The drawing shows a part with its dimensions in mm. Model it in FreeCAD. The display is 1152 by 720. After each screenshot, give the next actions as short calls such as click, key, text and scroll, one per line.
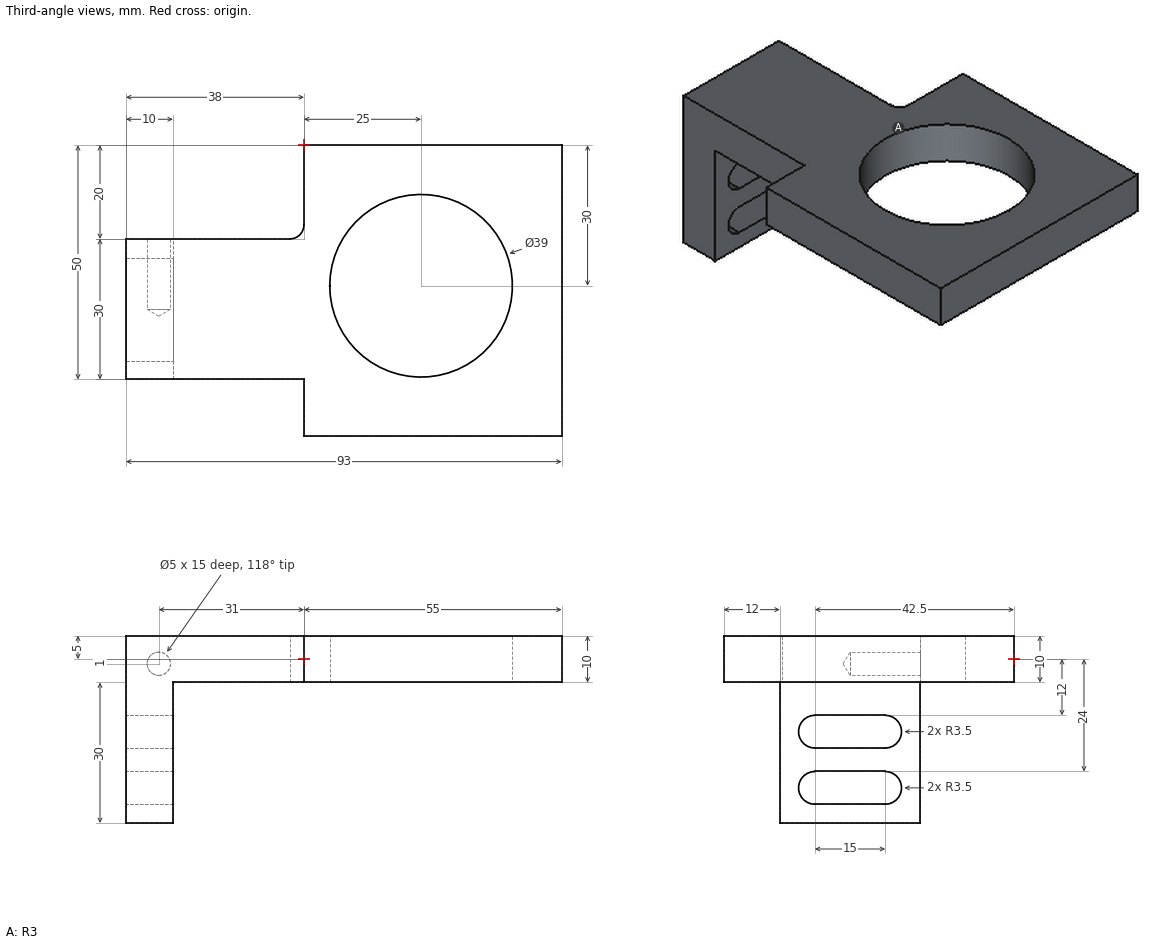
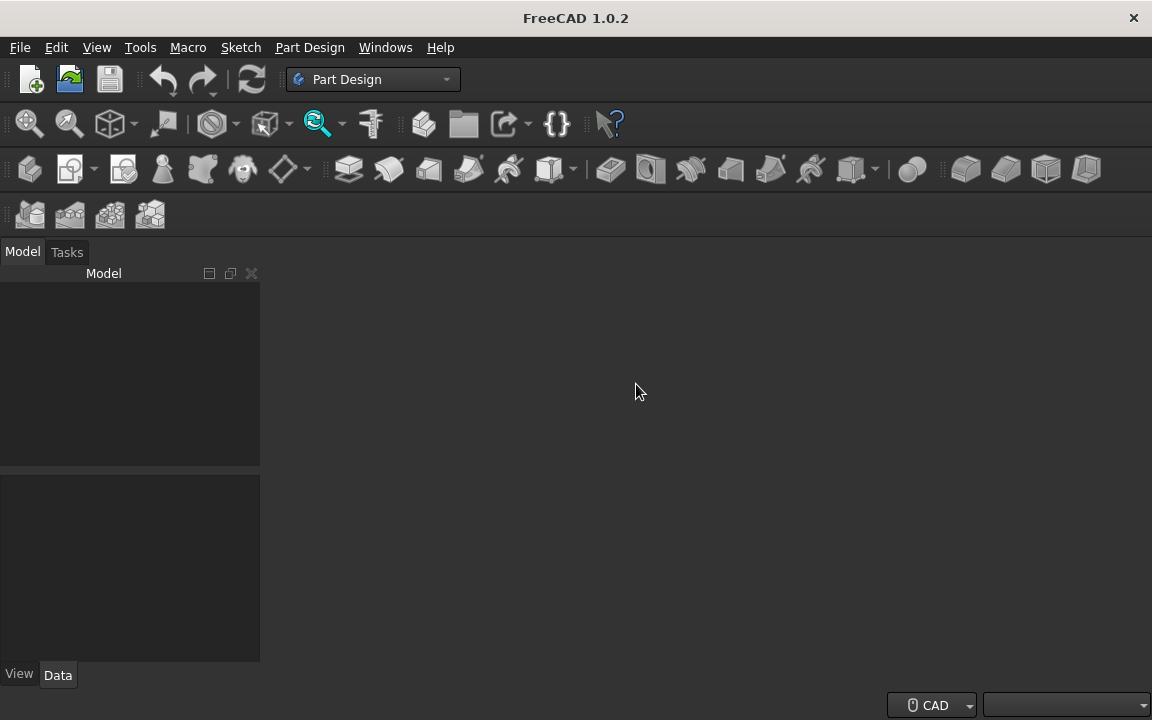
key(ctrl+n)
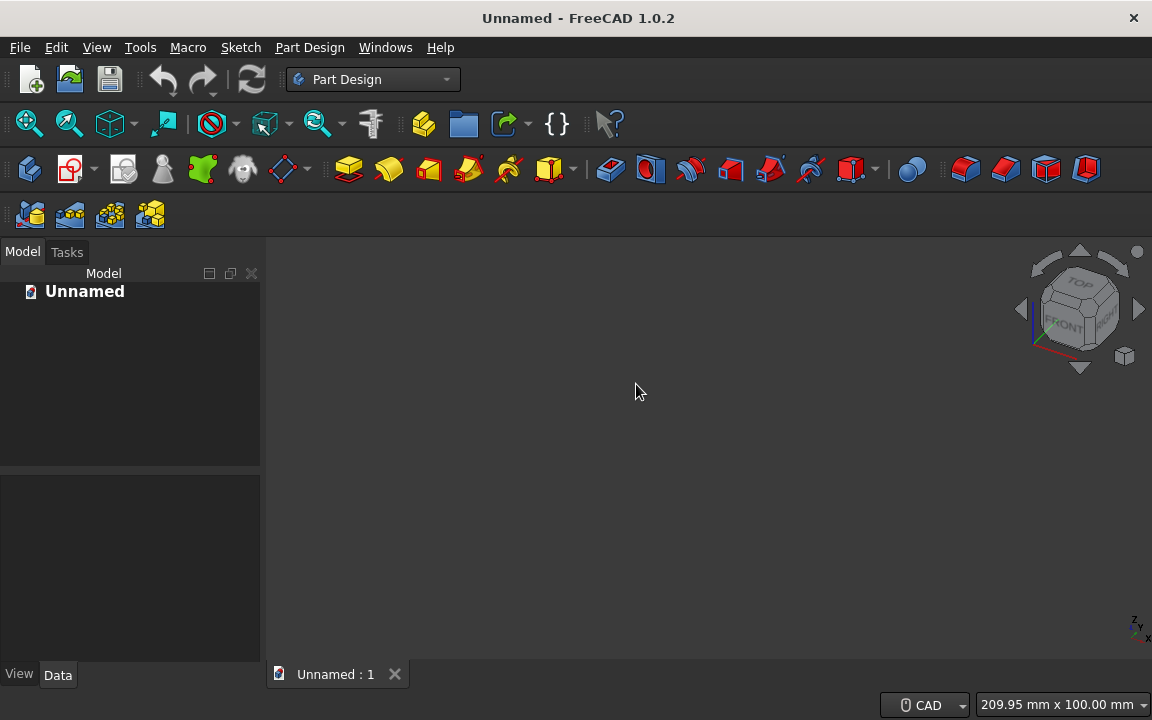
click(70, 170)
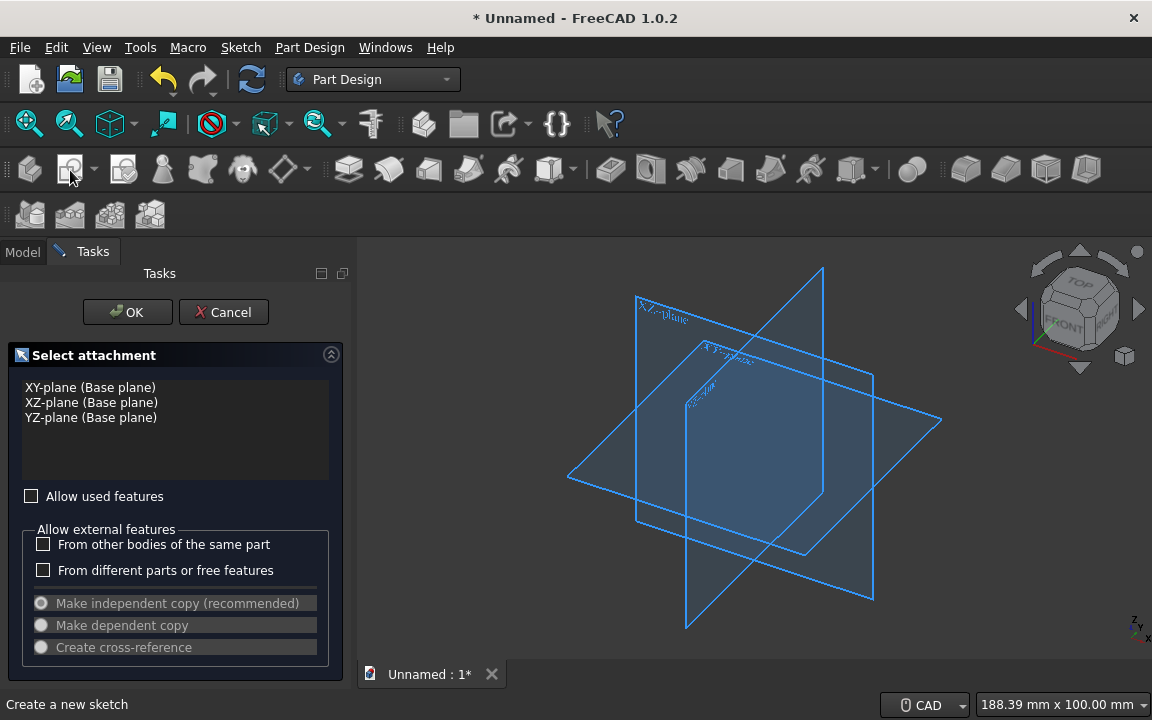
click(82, 388)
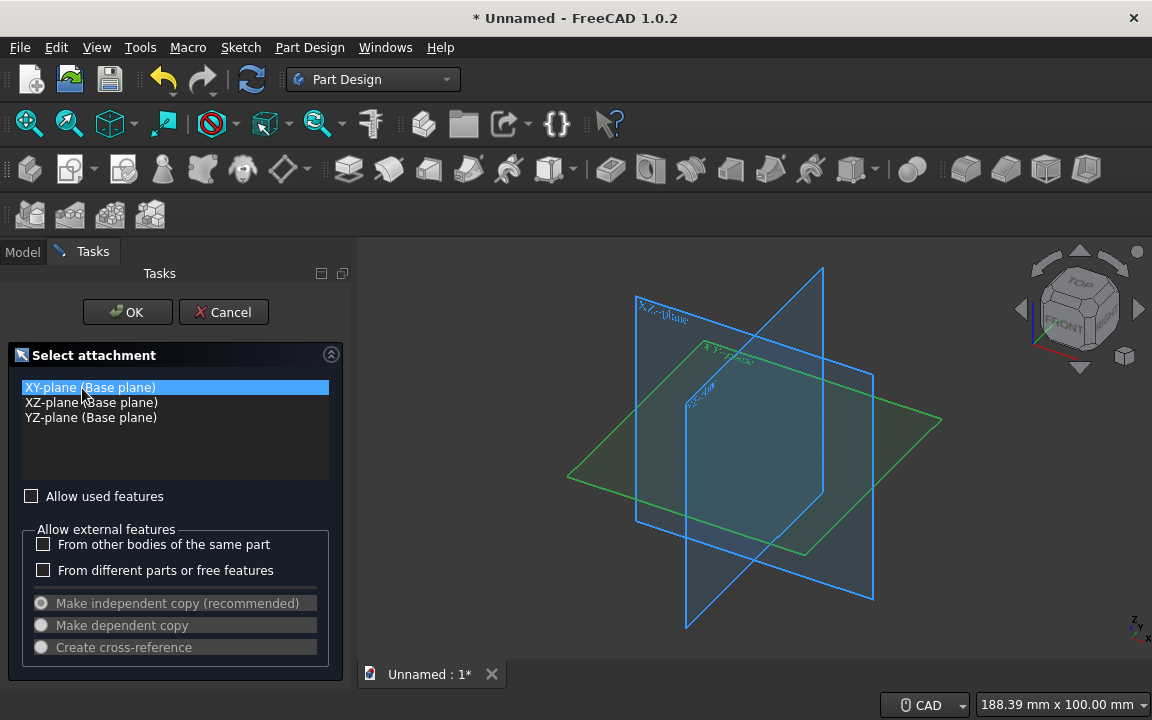
click(128, 312)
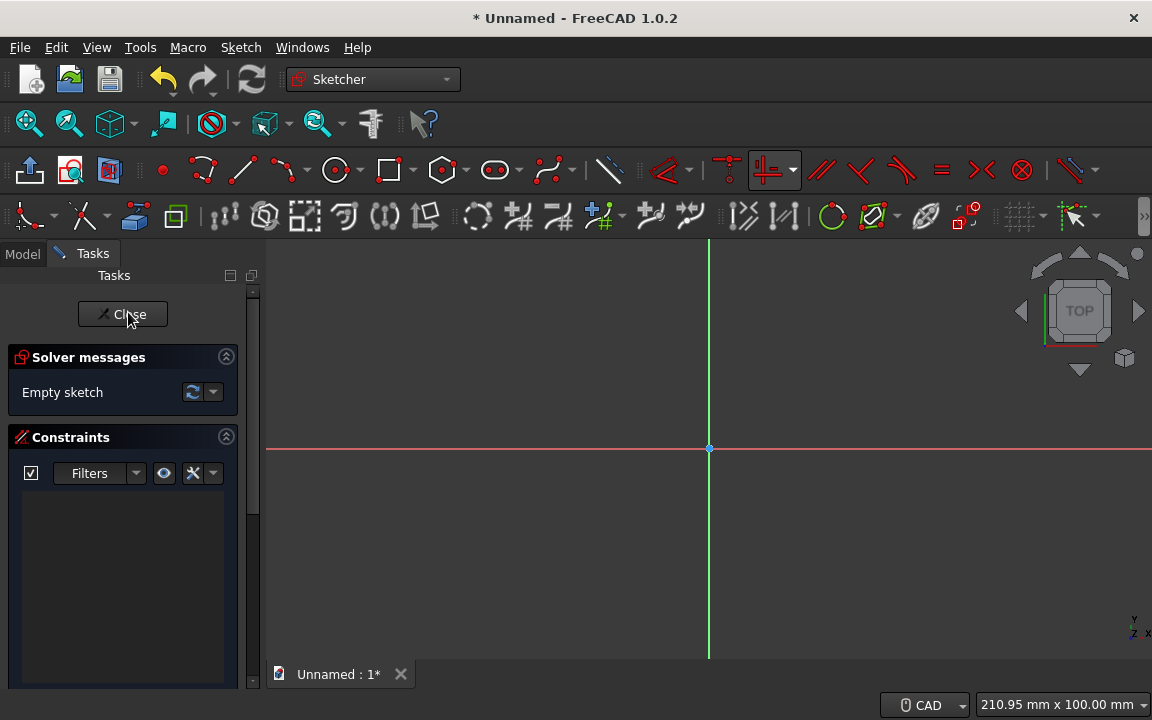
scroll(294, 267, down, 1)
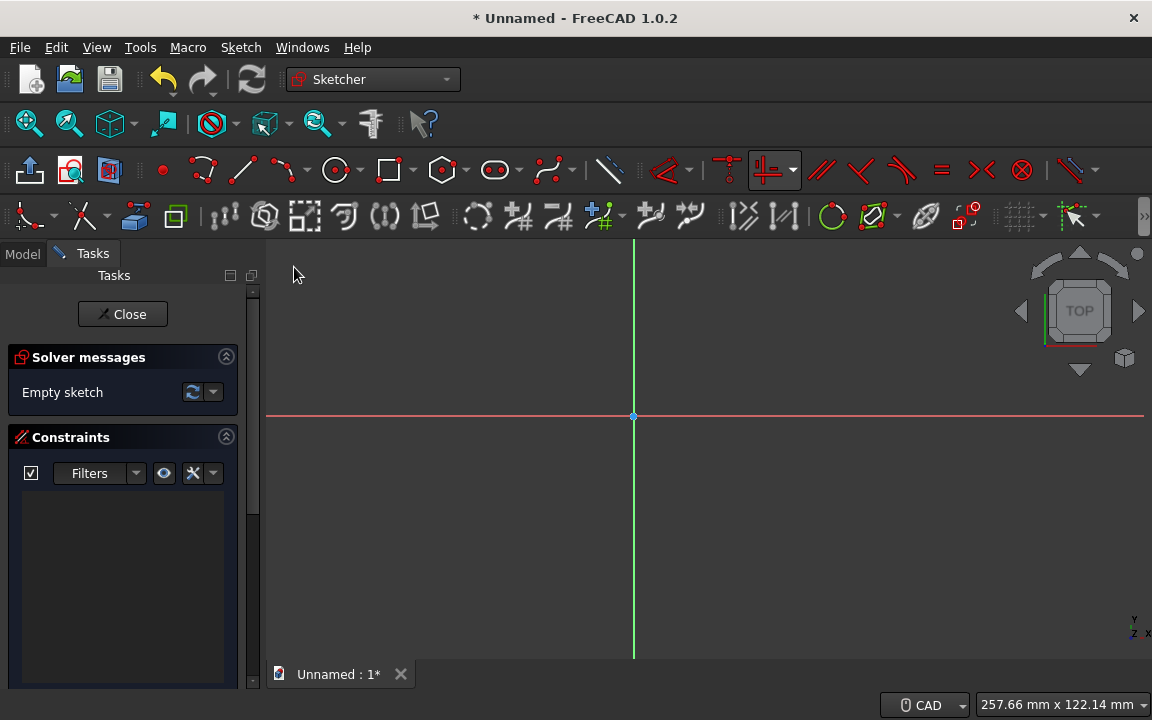
scroll(709, 610, up, 2)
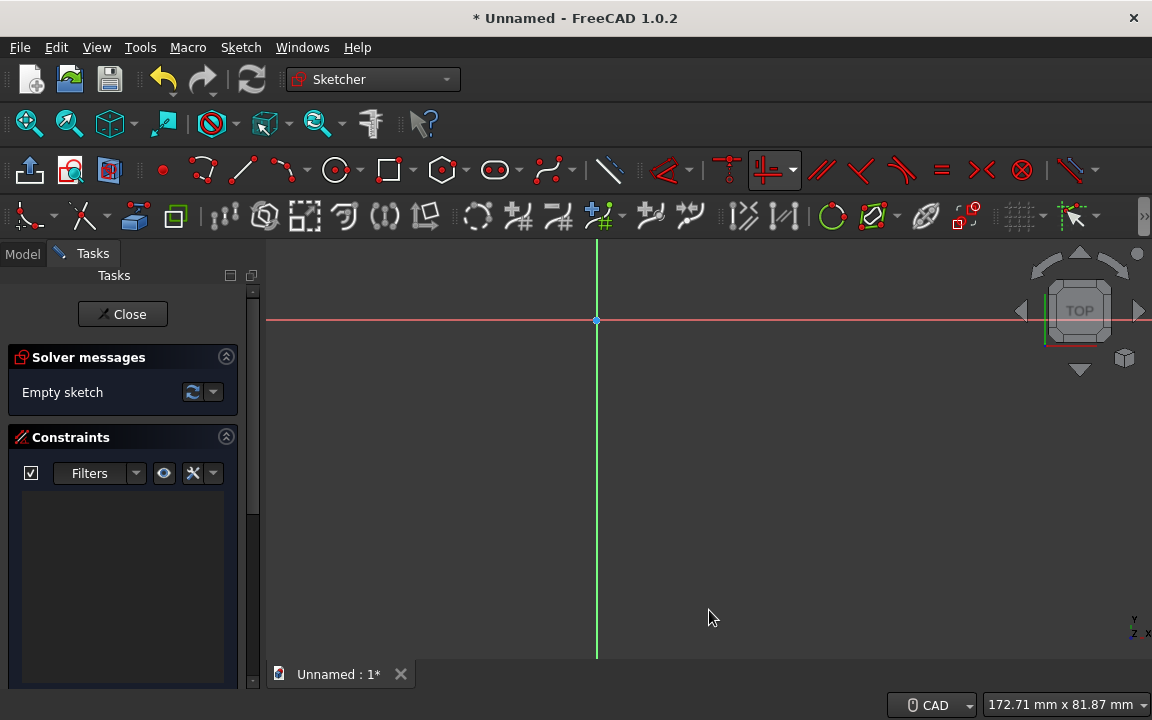
click(204, 170)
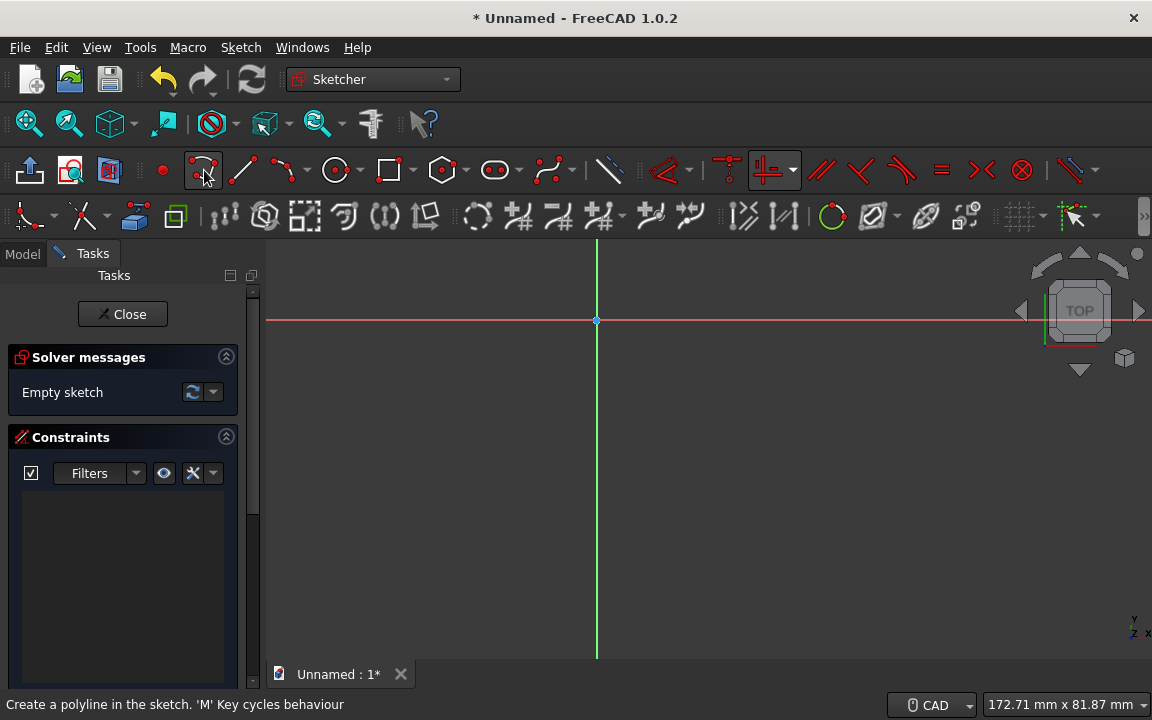
click(597, 320)
click(606, 423)
click(402, 423)
click(402, 577)
click(879, 577)
click(879, 329)
click(597, 320)
key(Escape)
key(Escape)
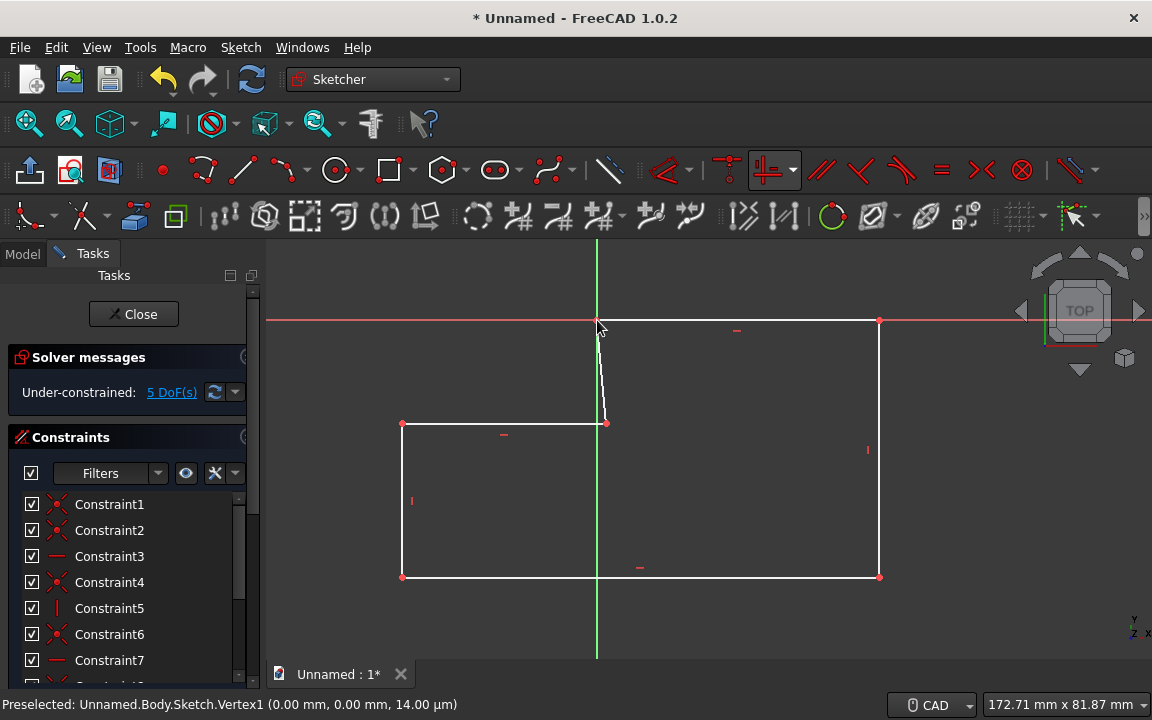
click(599, 351)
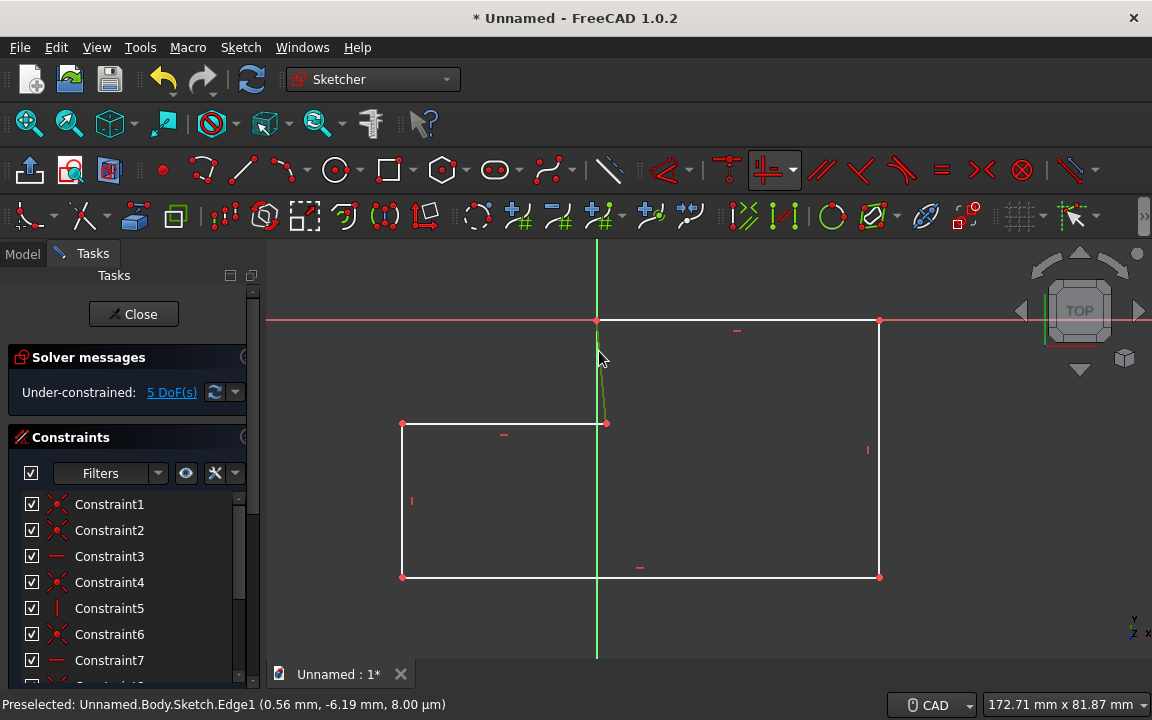
click(796, 170)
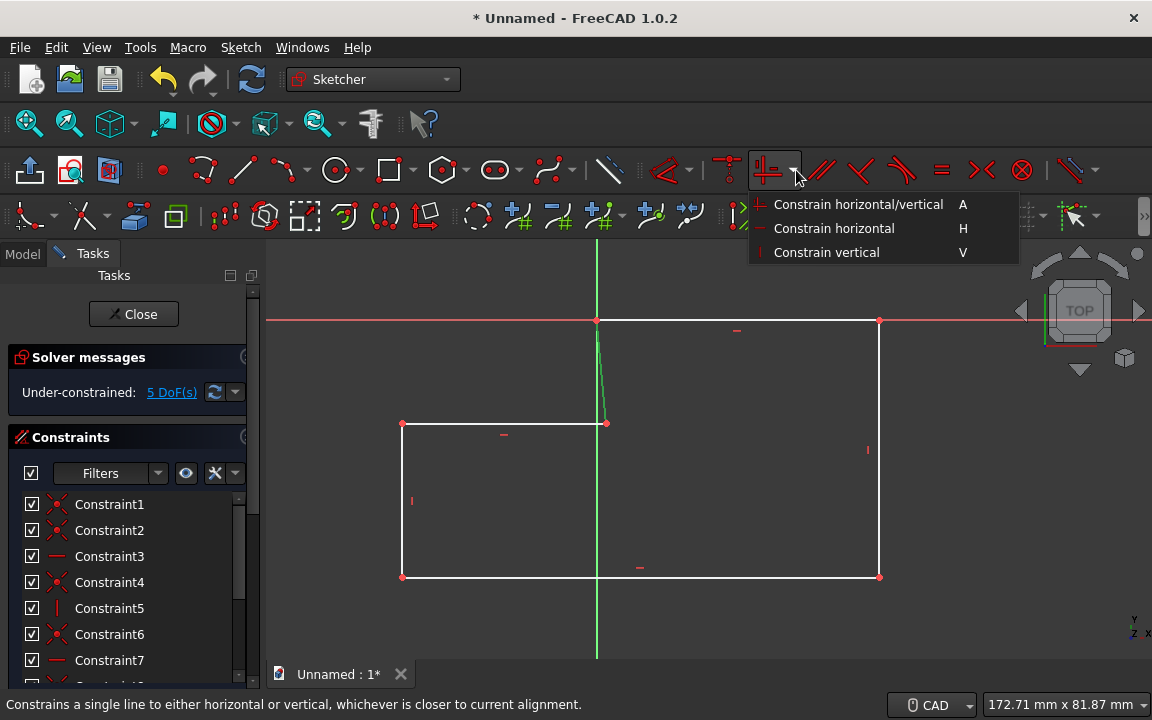
click(884, 252)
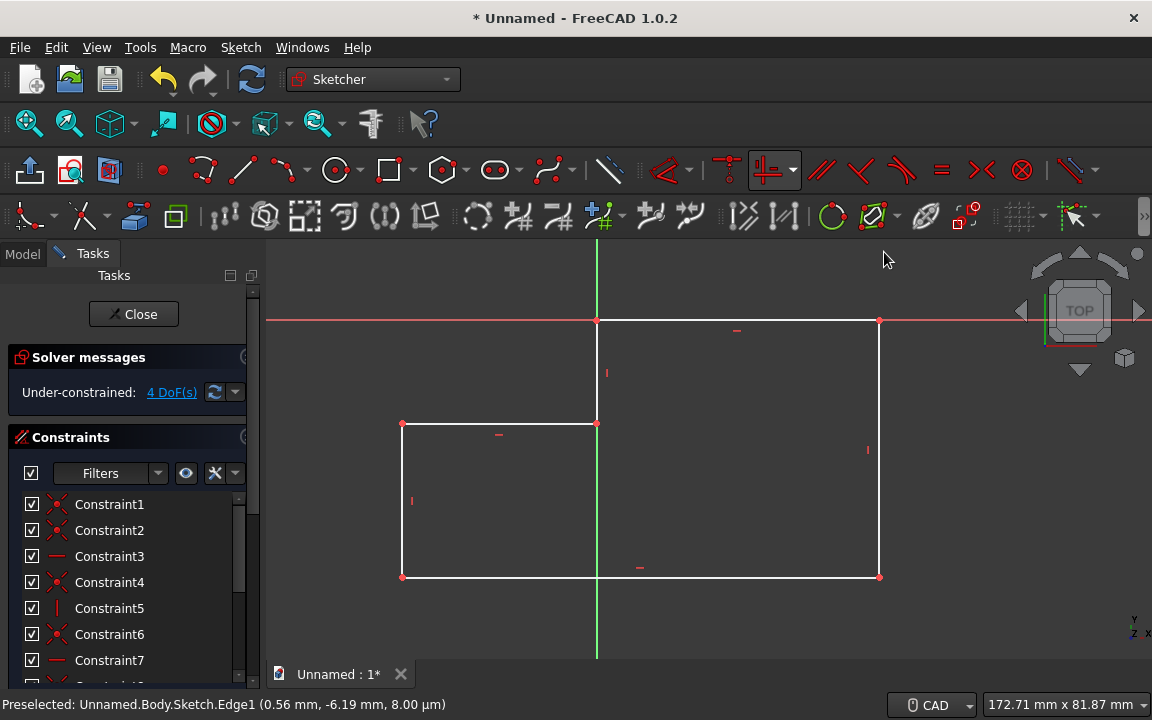
click(597, 351)